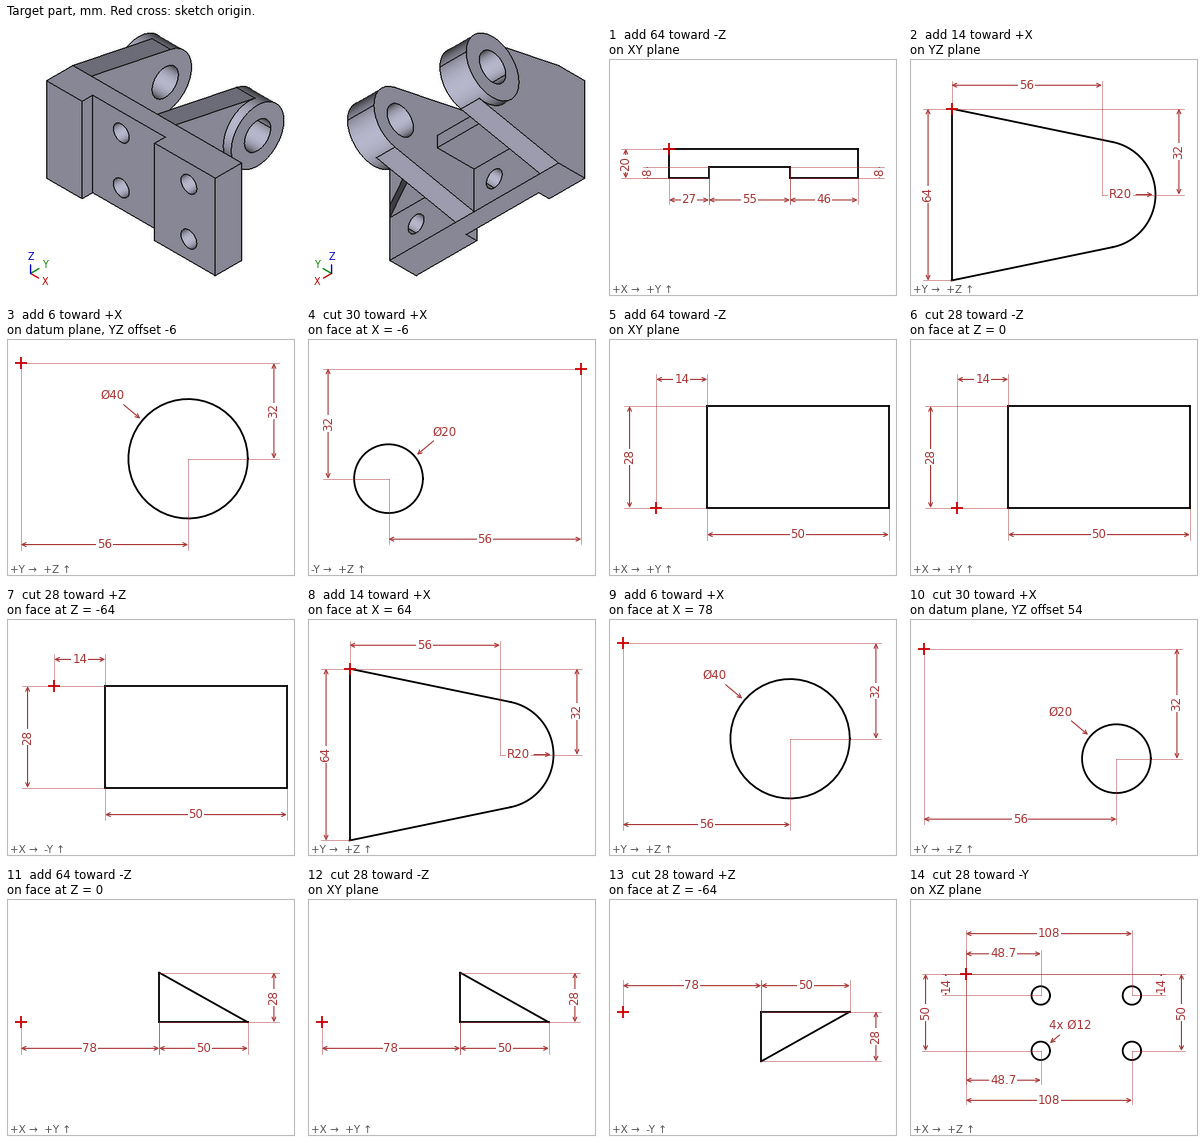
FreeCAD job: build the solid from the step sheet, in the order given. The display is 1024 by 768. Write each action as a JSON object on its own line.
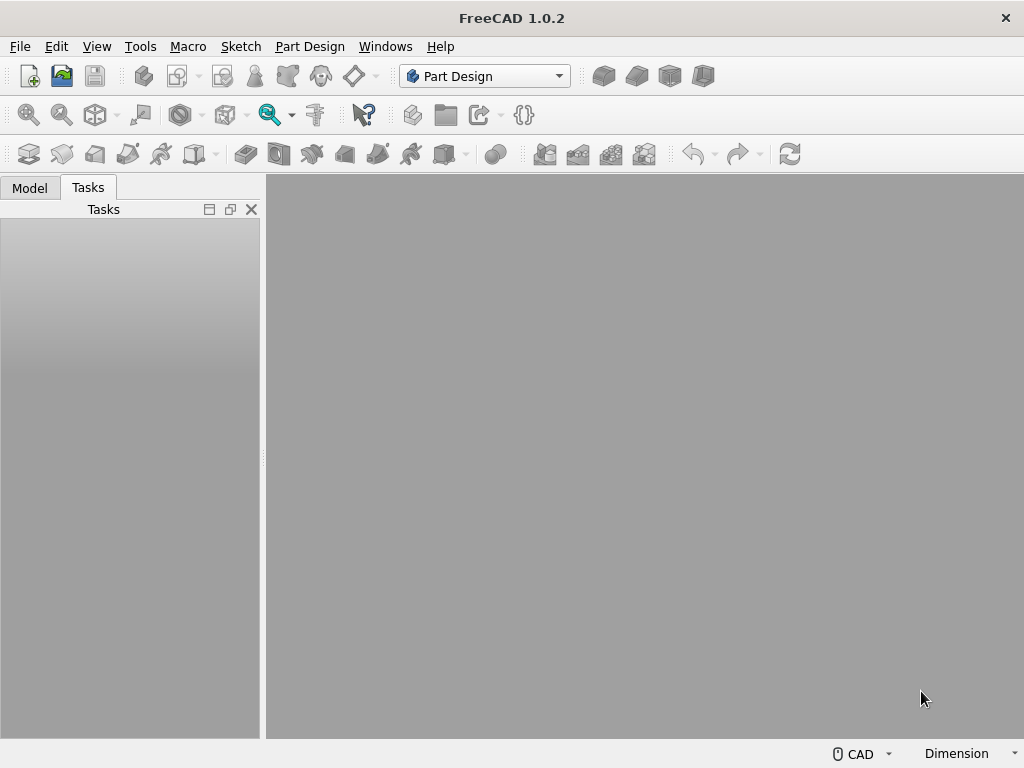
{"action": "left_click", "coordinate": [29, 76]}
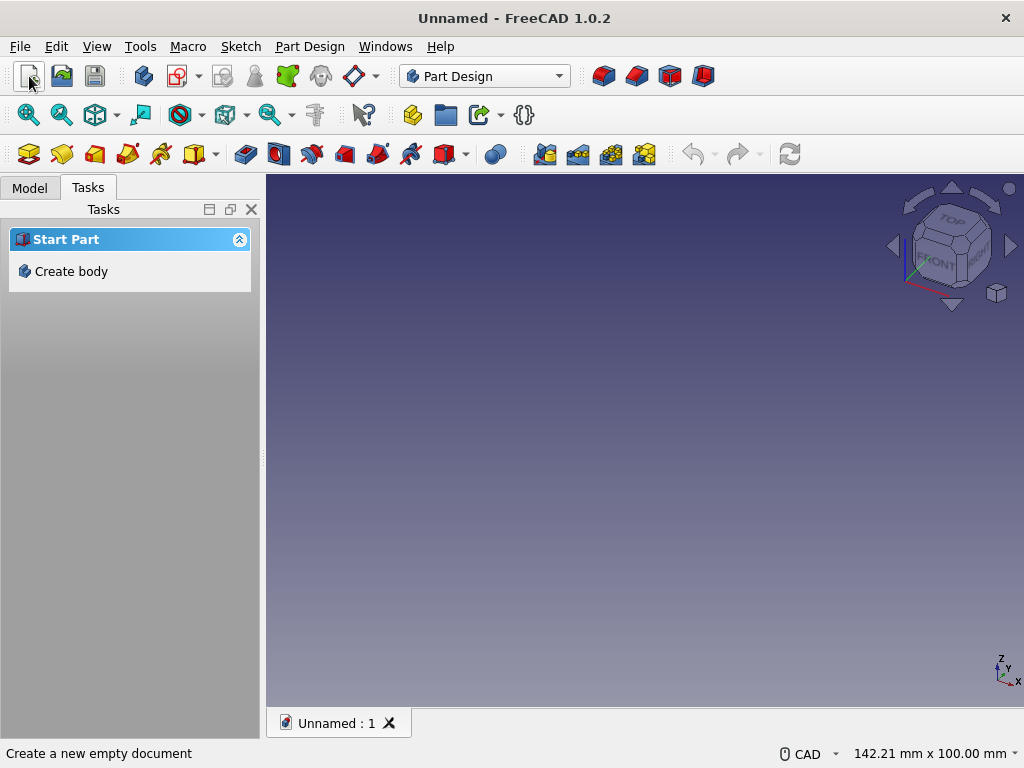
{"action": "left_click", "coordinate": [176, 76]}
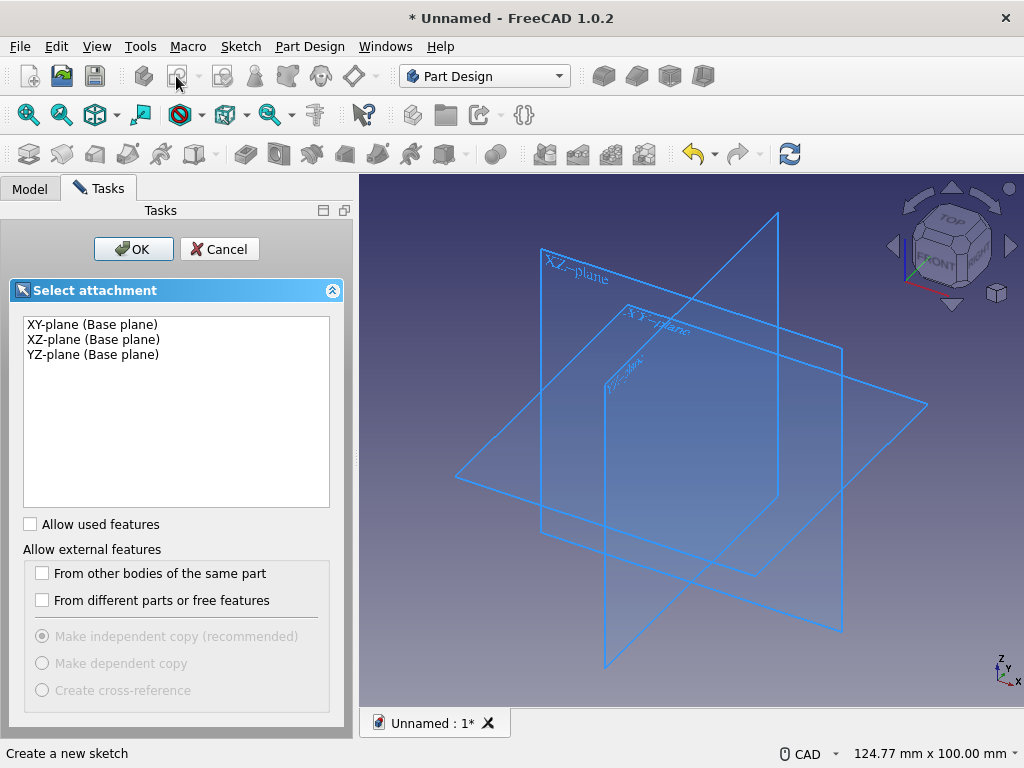
{"action": "left_click", "coordinate": [84, 324]}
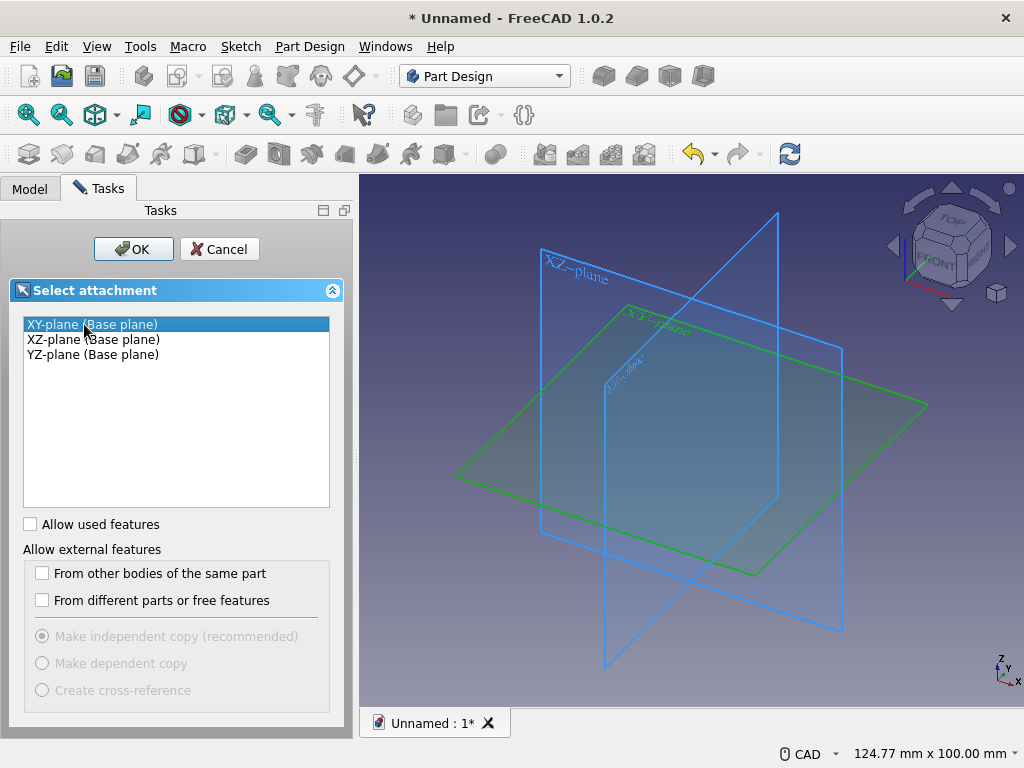
{"action": "left_click", "coordinate": [134, 249]}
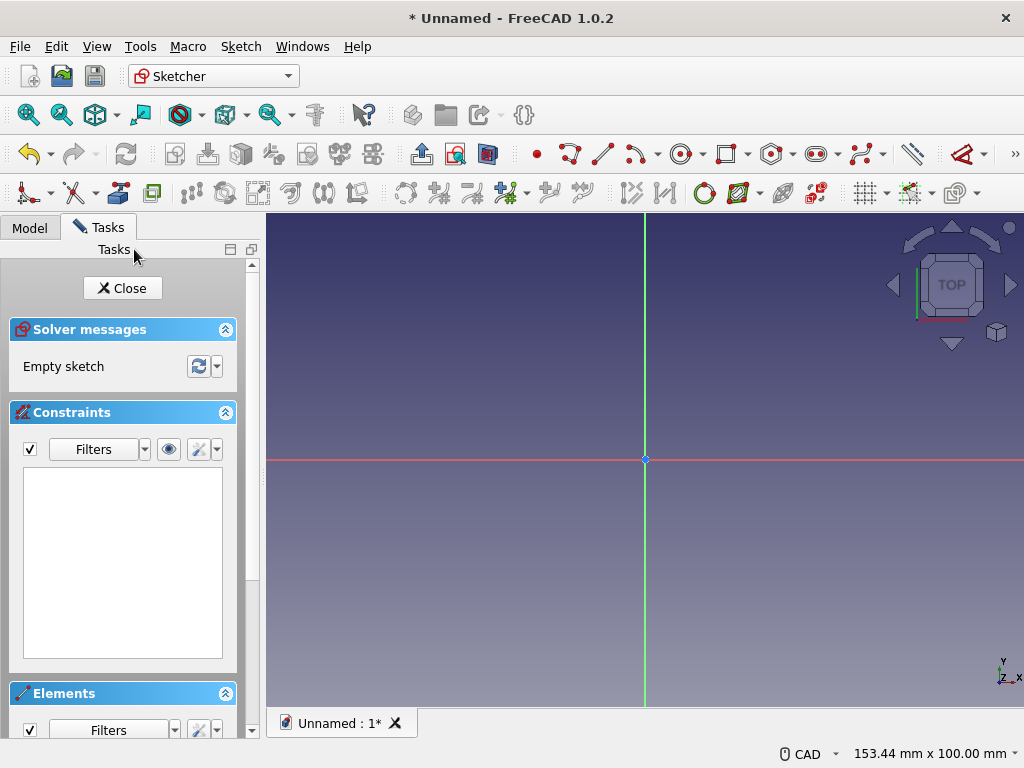
{"action": "scroll", "coordinate": [294, 400], "scroll_direction": "down", "scroll_amount": 3}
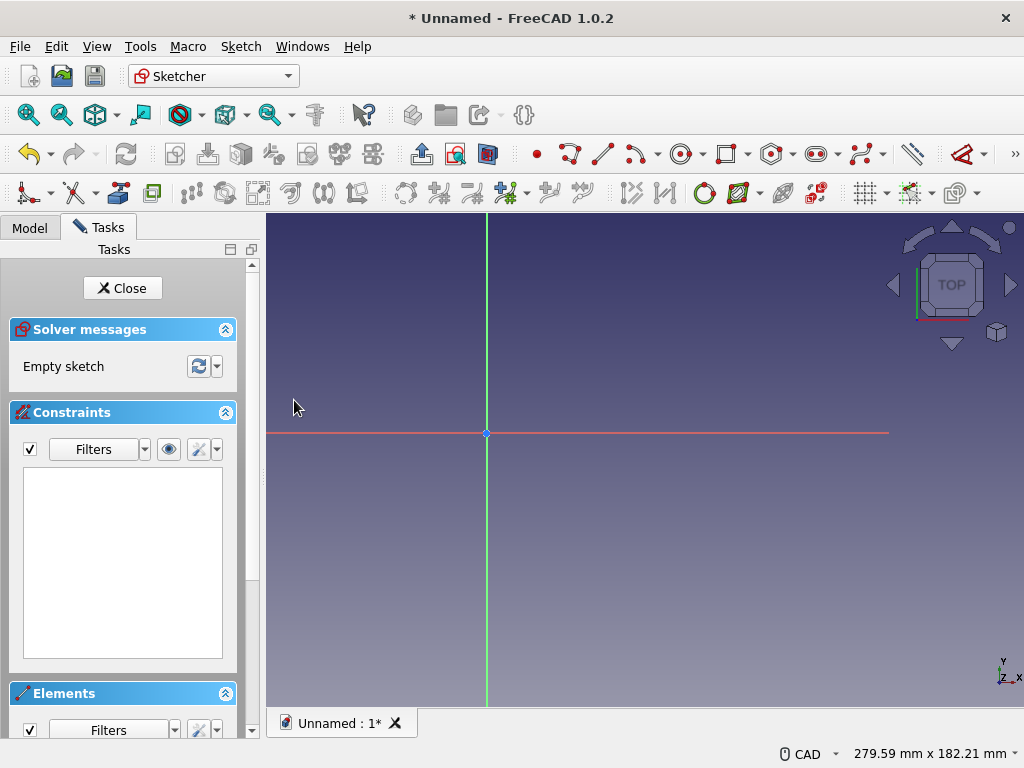
{"action": "left_click", "coordinate": [570, 154]}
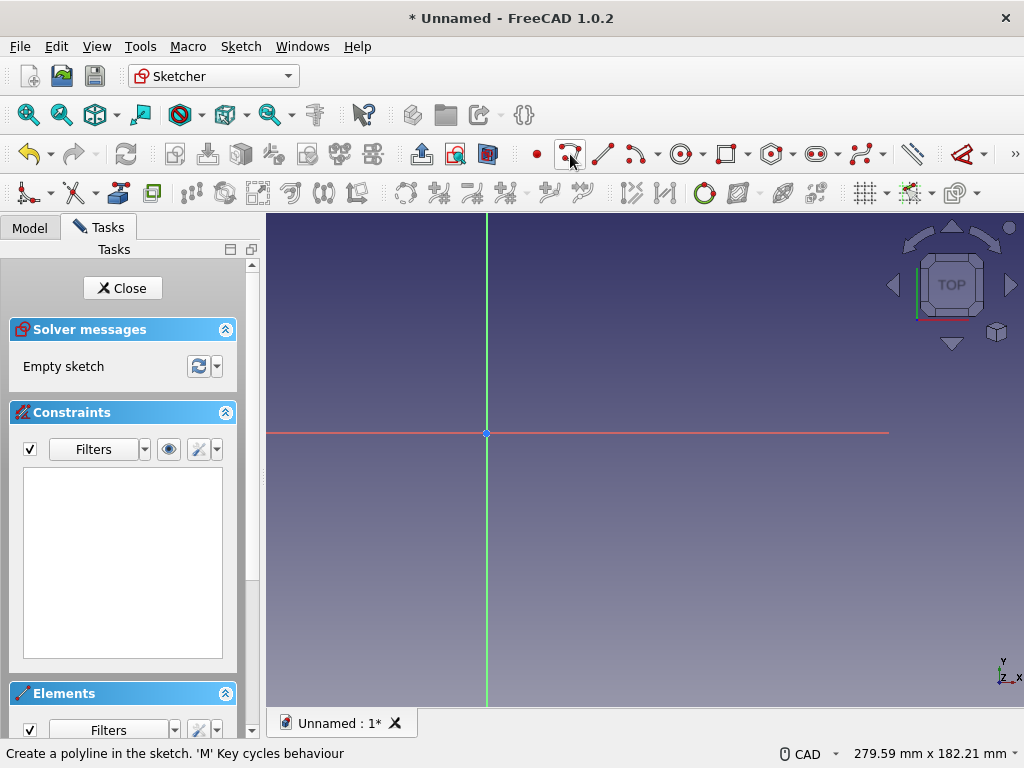
{"action": "left_click", "coordinate": [487, 433]}
{"action": "left_click", "coordinate": [496, 487]}
{"action": "left_click", "coordinate": [560, 487]}
{"action": "left_click", "coordinate": [560, 466]}
{"action": "left_click", "coordinate": [709, 466]}
{"action": "left_click", "coordinate": [709, 487]}
{"action": "left_click", "coordinate": [834, 487]}
{"action": "left_click", "coordinate": [834, 442]}
{"action": "left_click", "coordinate": [487, 433]}
{"action": "key", "text": "Escape"}
{"action": "key", "text": "Escape"}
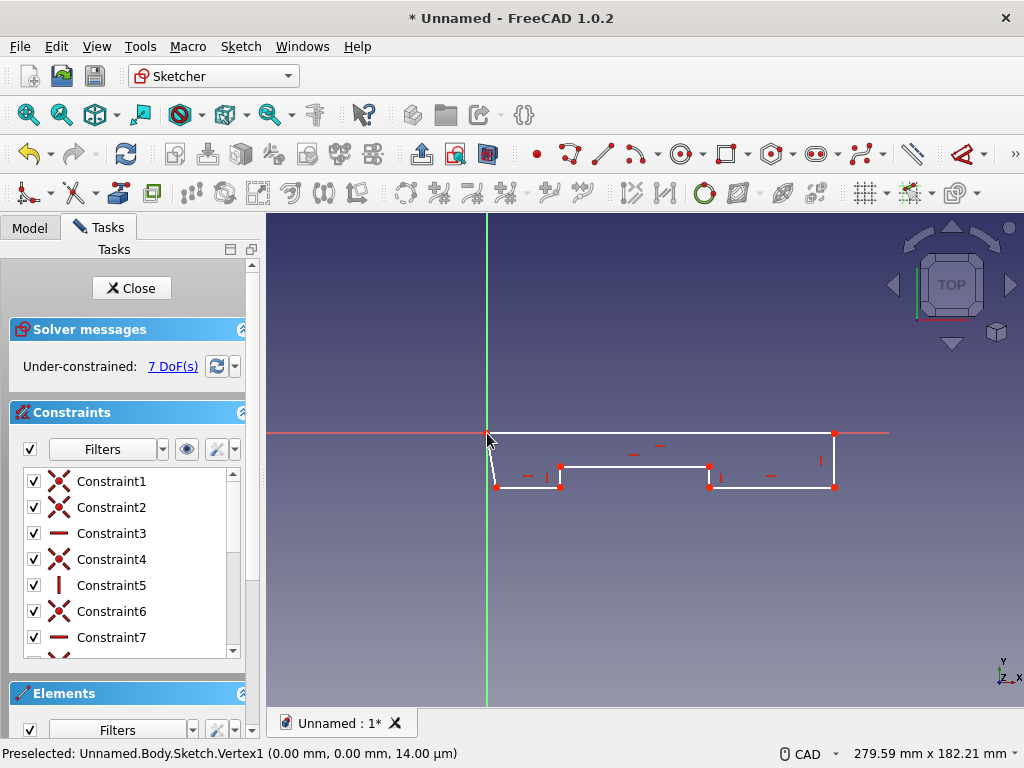
{"action": "left_click", "coordinate": [489, 450]}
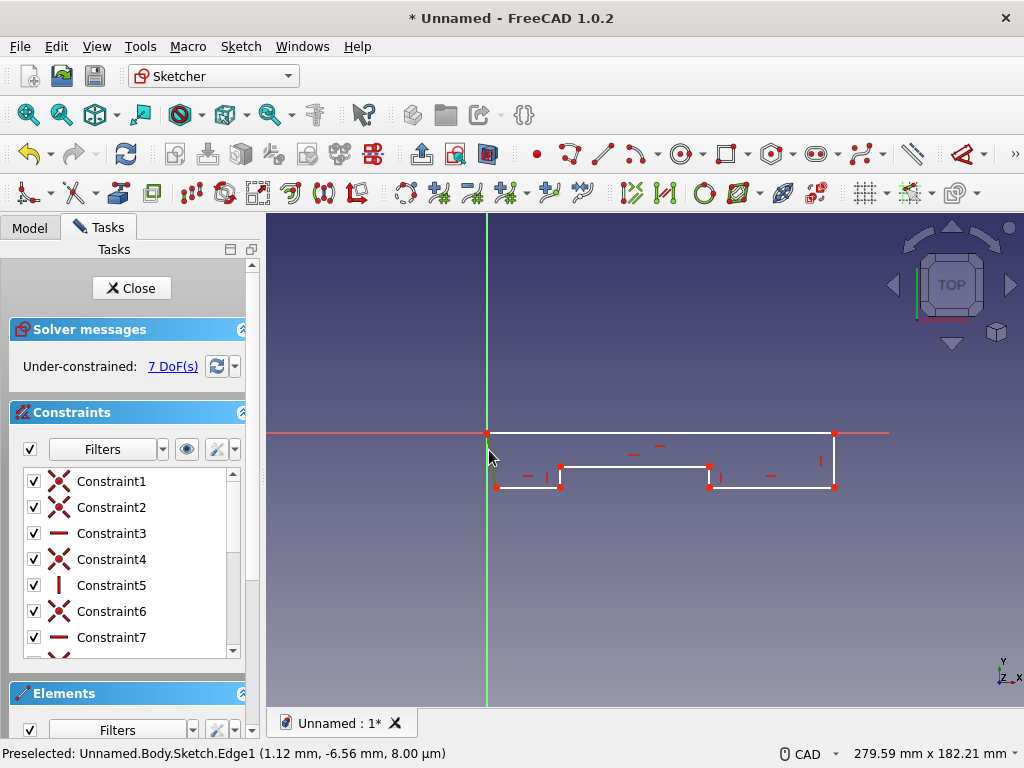
{"action": "key", "text": "v"}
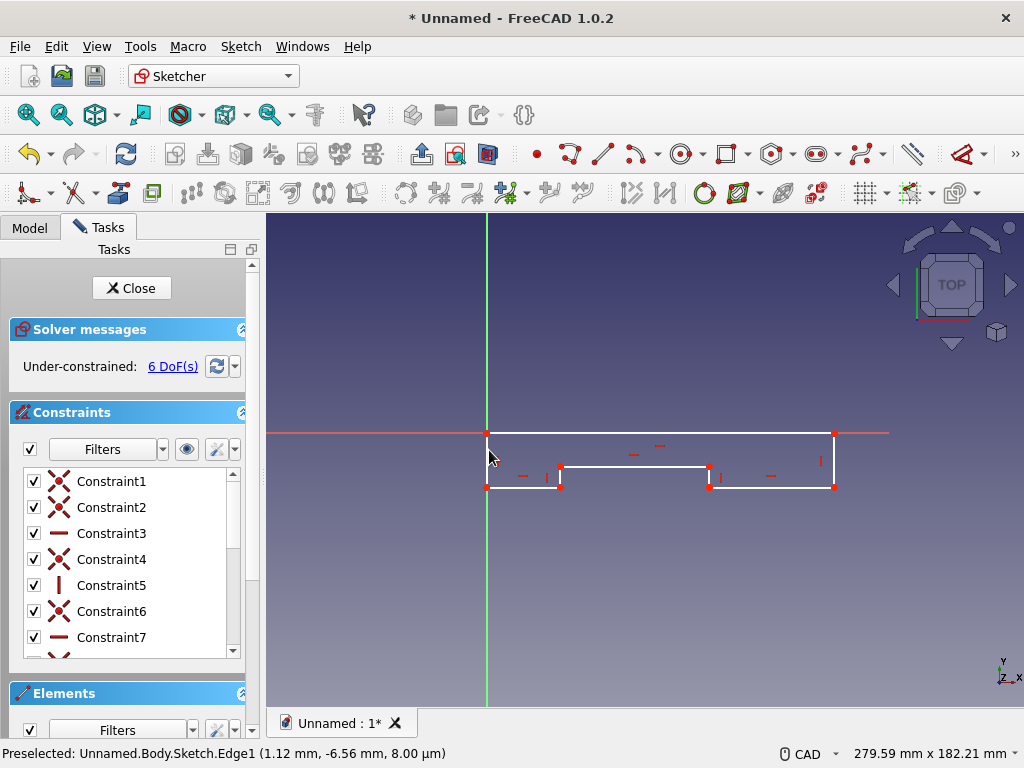
{"action": "left_click", "coordinate": [962, 154]}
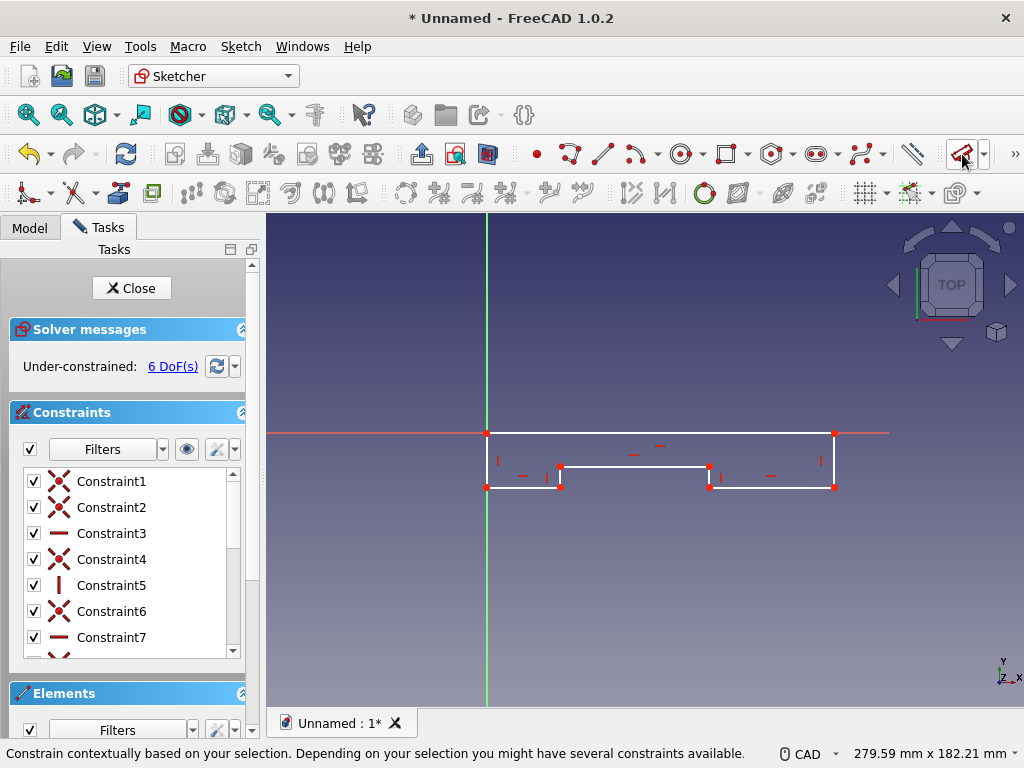
{"action": "scroll", "coordinate": [560, 478], "scroll_direction": "up", "scroll_amount": 4}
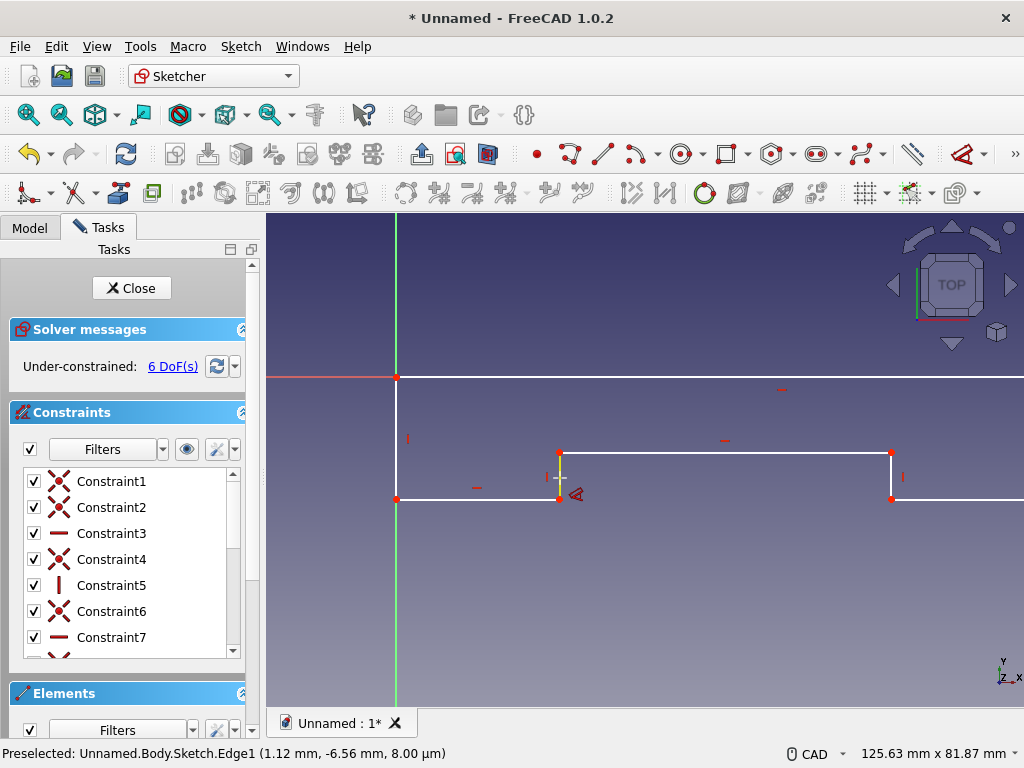
{"action": "left_click", "coordinate": [560, 476]}
{"action": "left_click", "coordinate": [526, 476]}